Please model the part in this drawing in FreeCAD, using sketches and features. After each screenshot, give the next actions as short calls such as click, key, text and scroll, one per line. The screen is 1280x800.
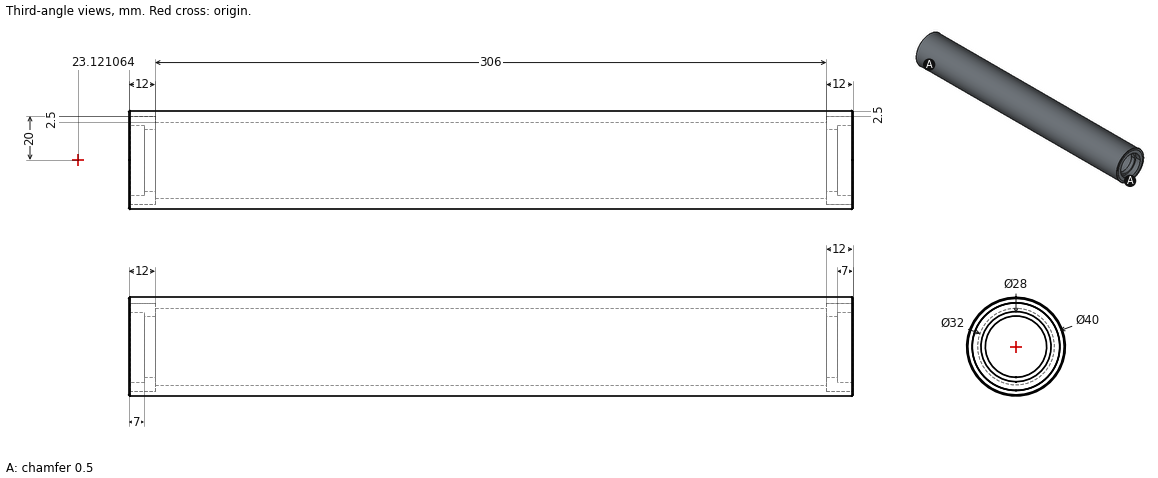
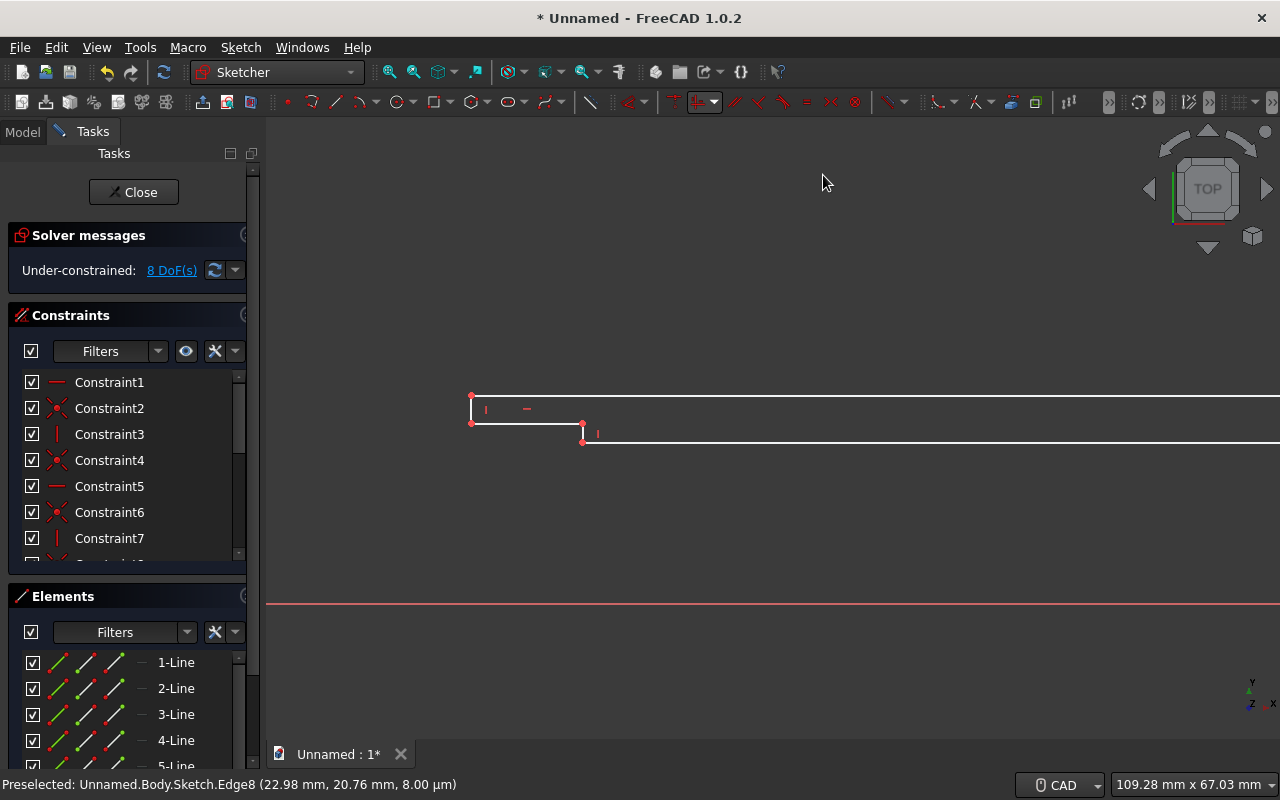
click(505, 424)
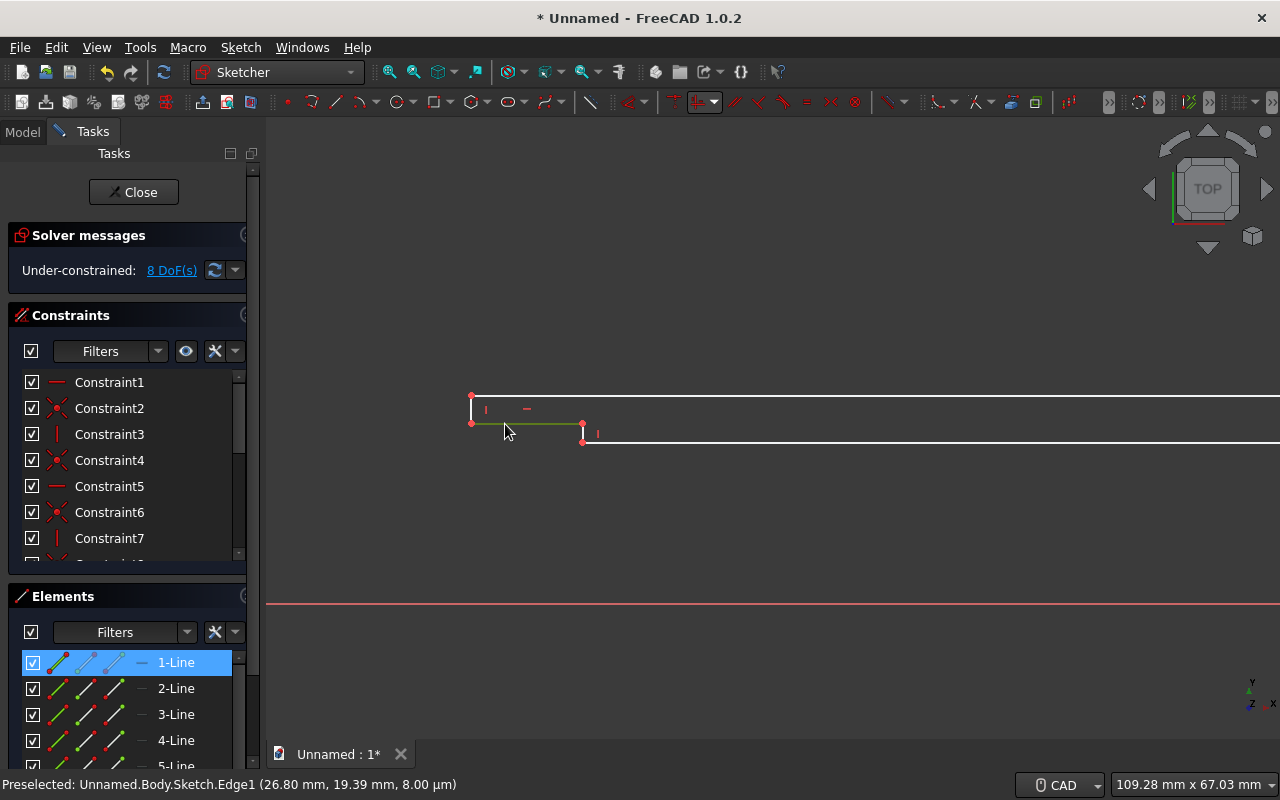
click(646, 102)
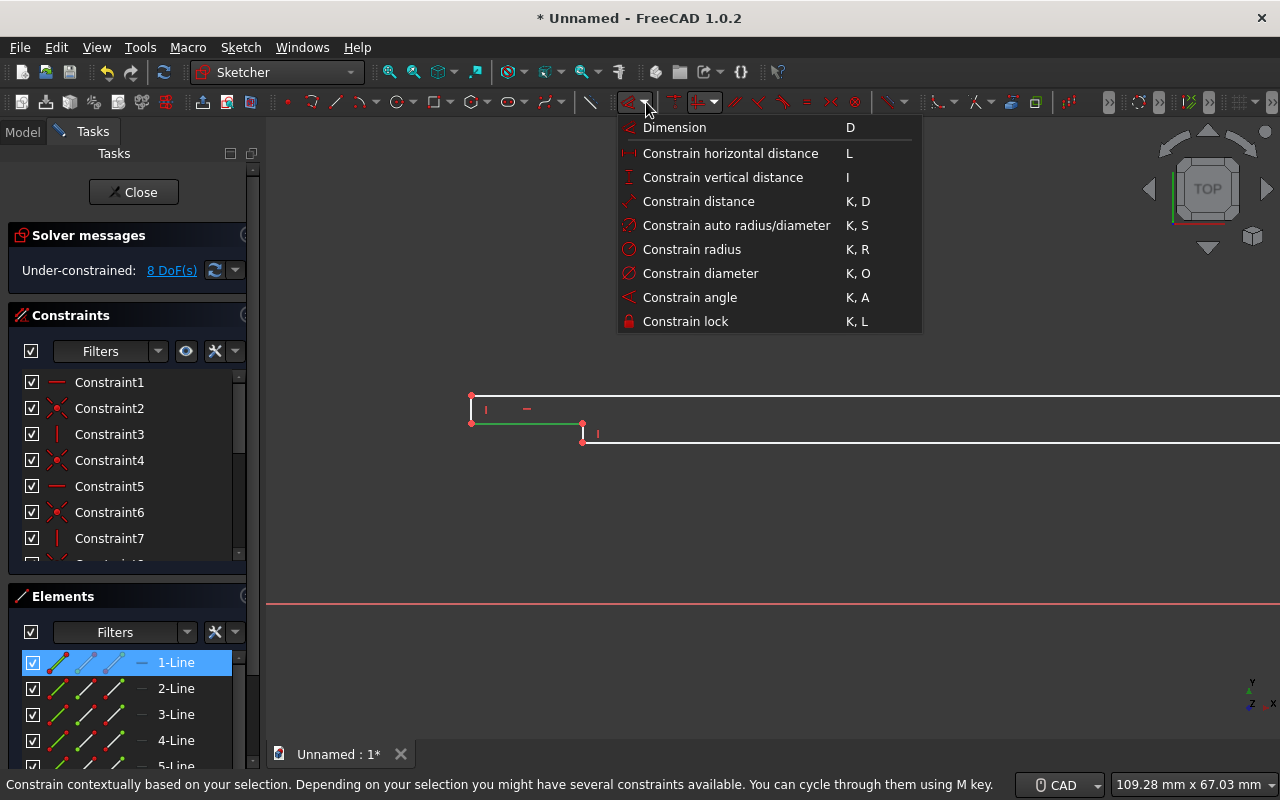
click(770, 153)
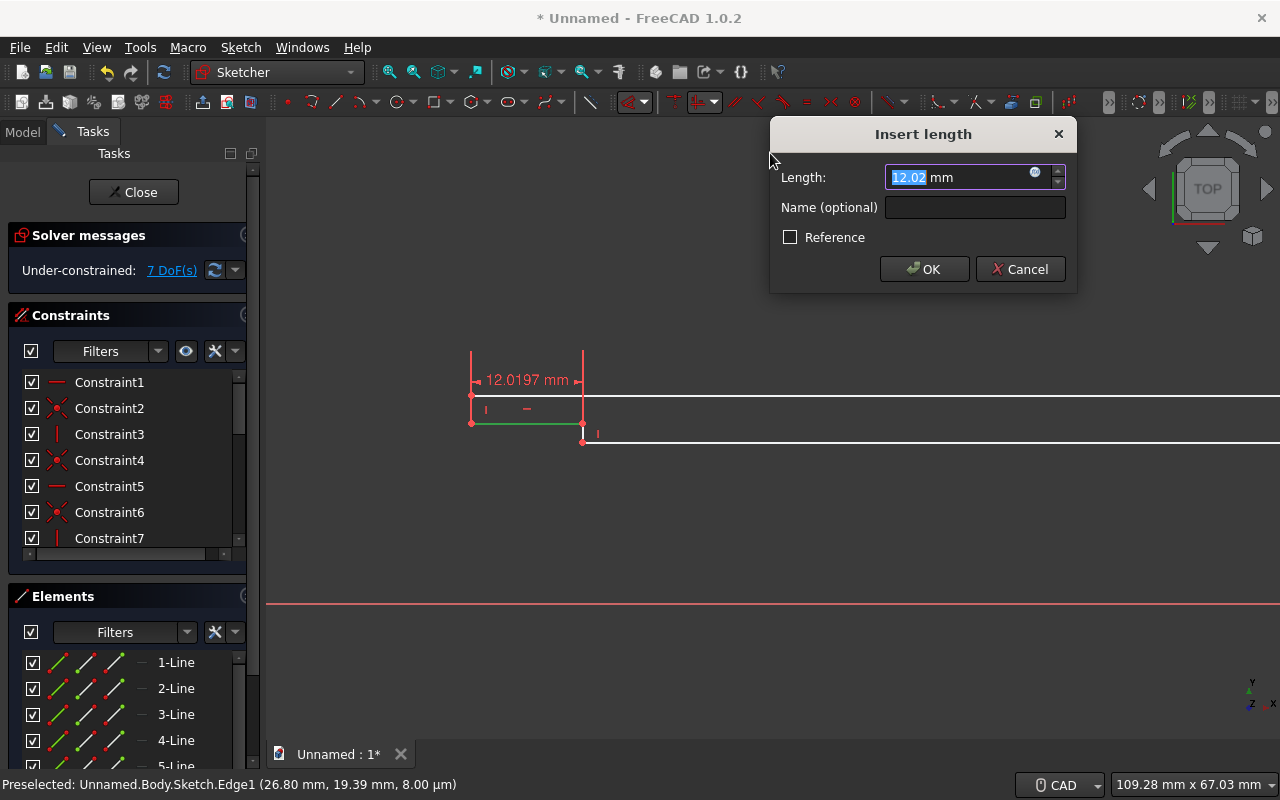
text(12)
key(Return)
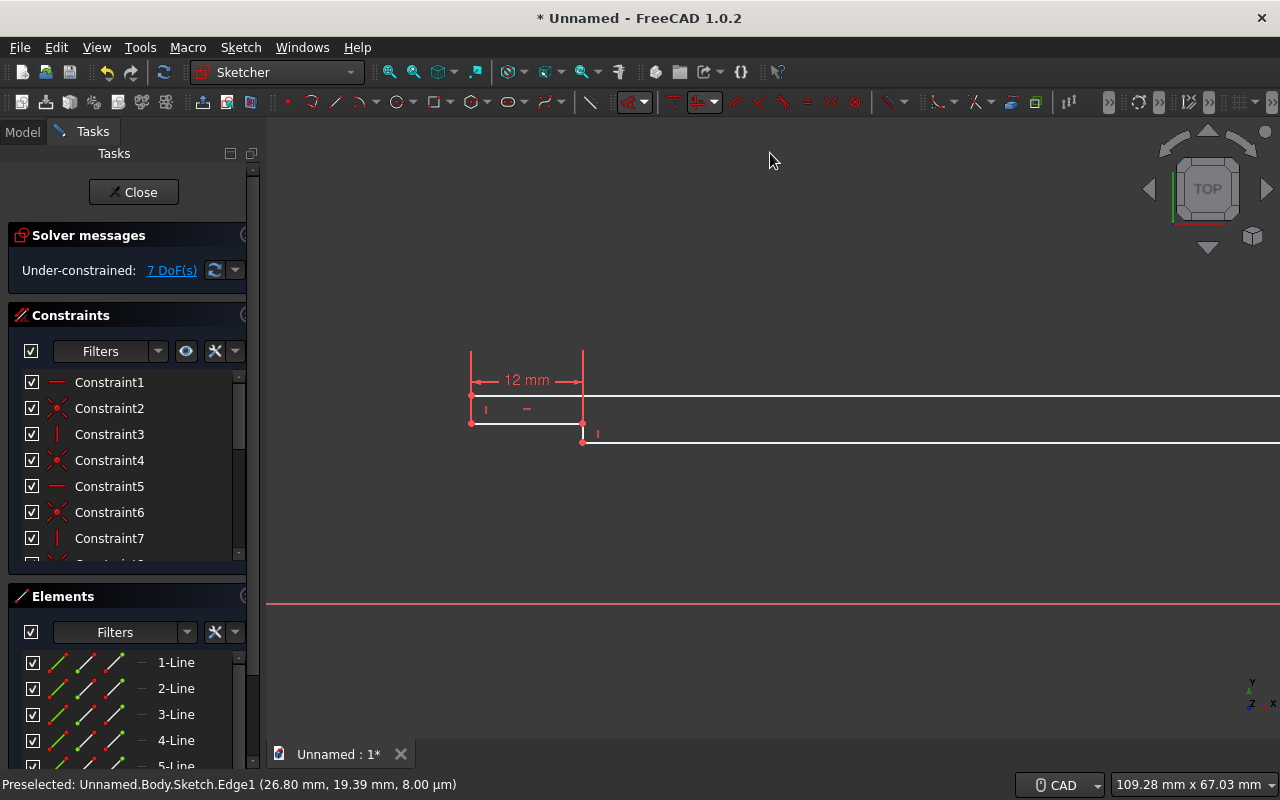
scroll(469, 414, down, 9)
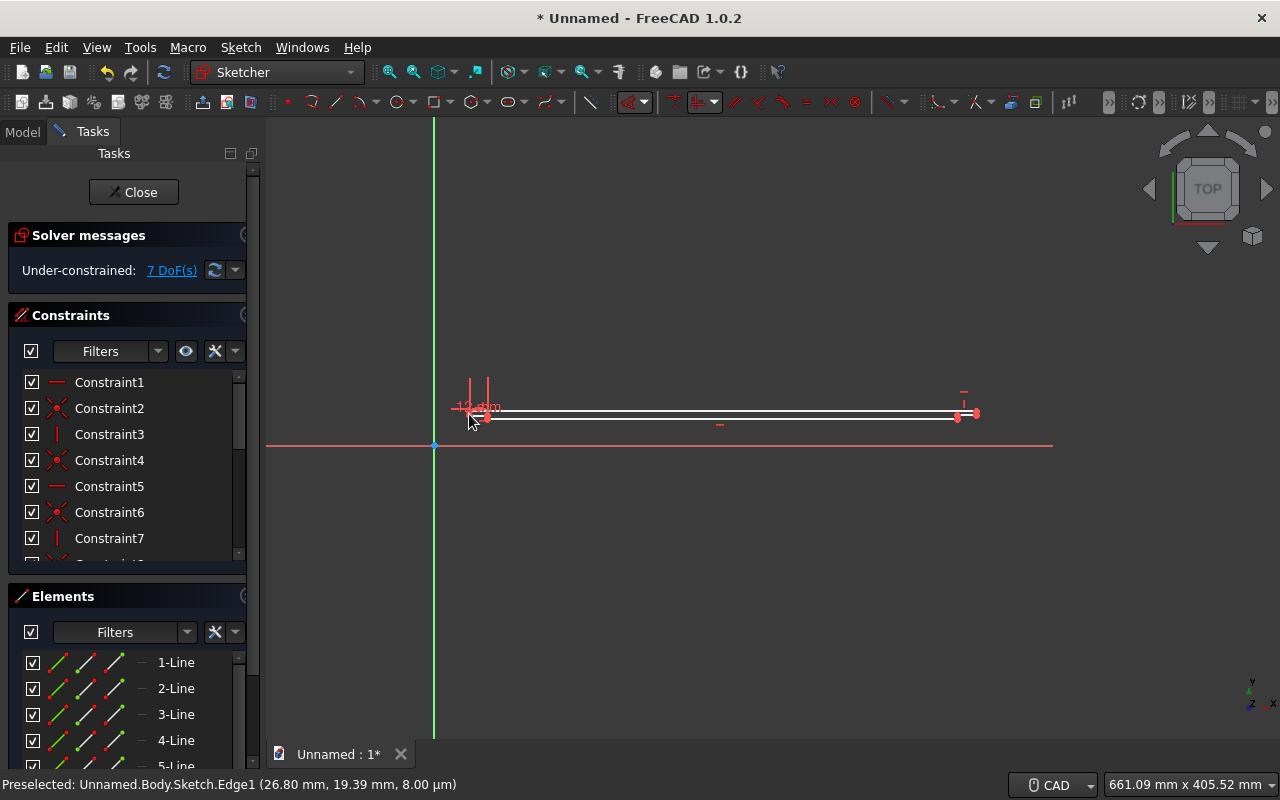
scroll(963, 415, up, 7)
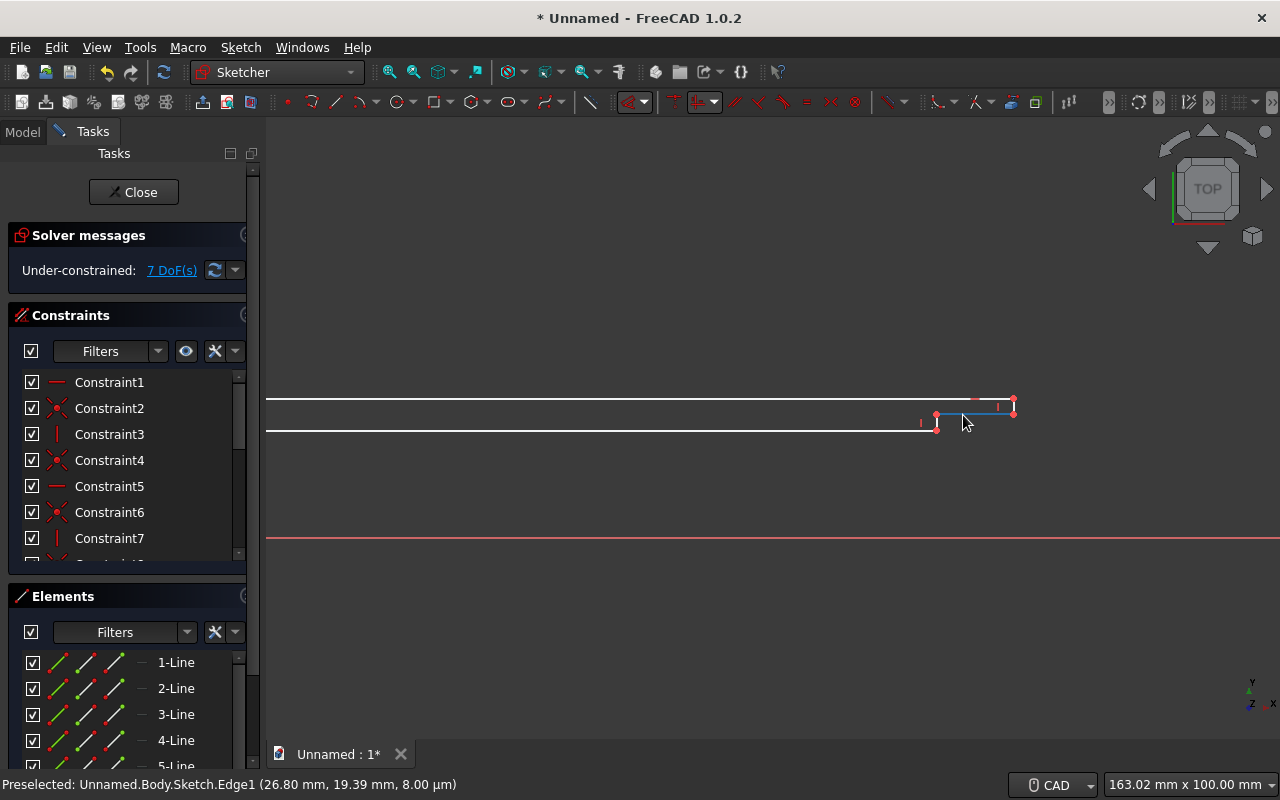
click(960, 414)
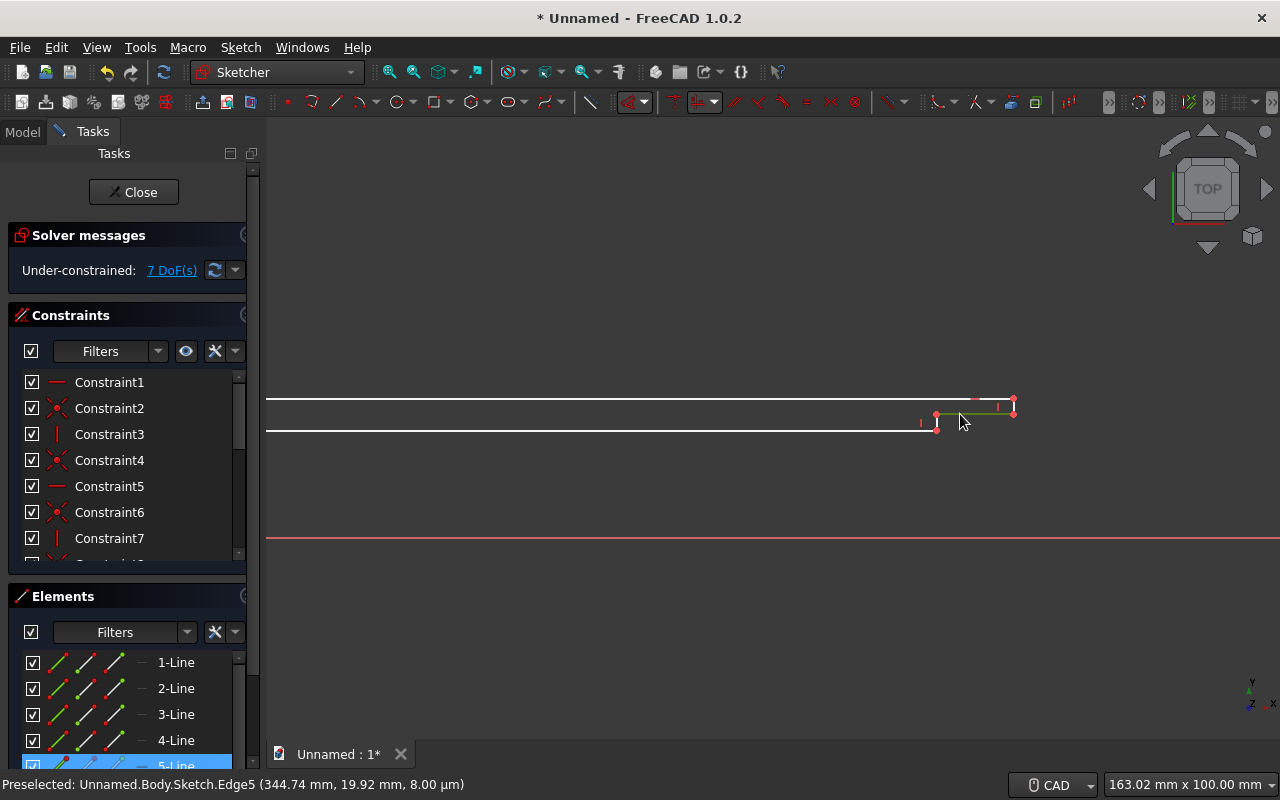
key(l)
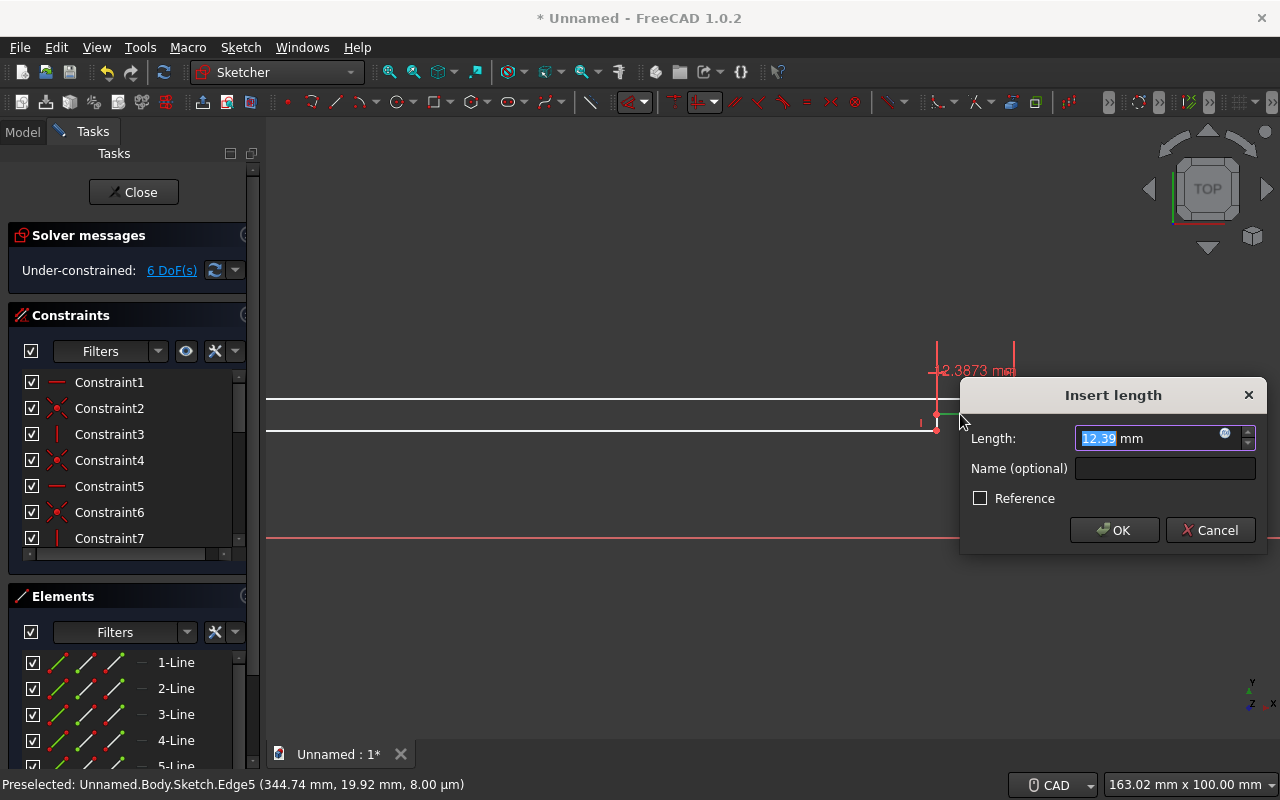
text(12)
key(Return)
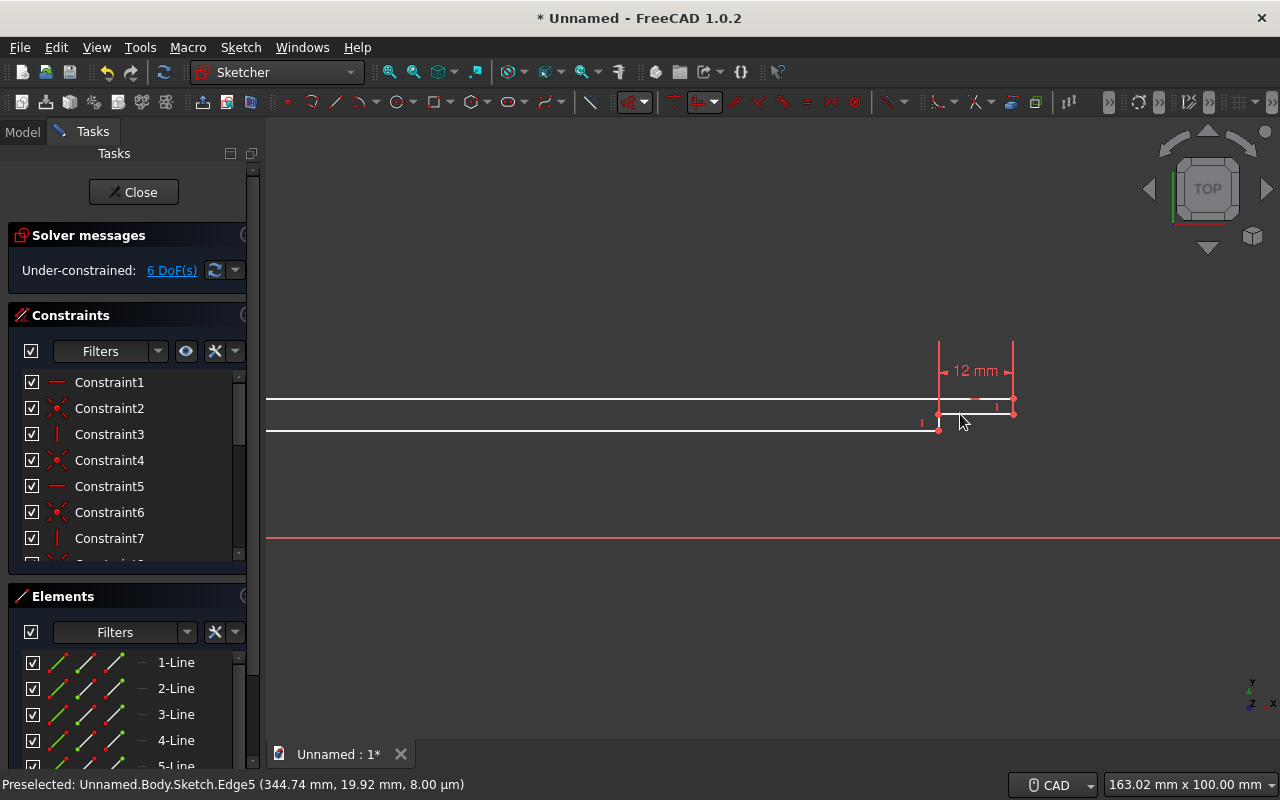
scroll(963, 415, down, 7)